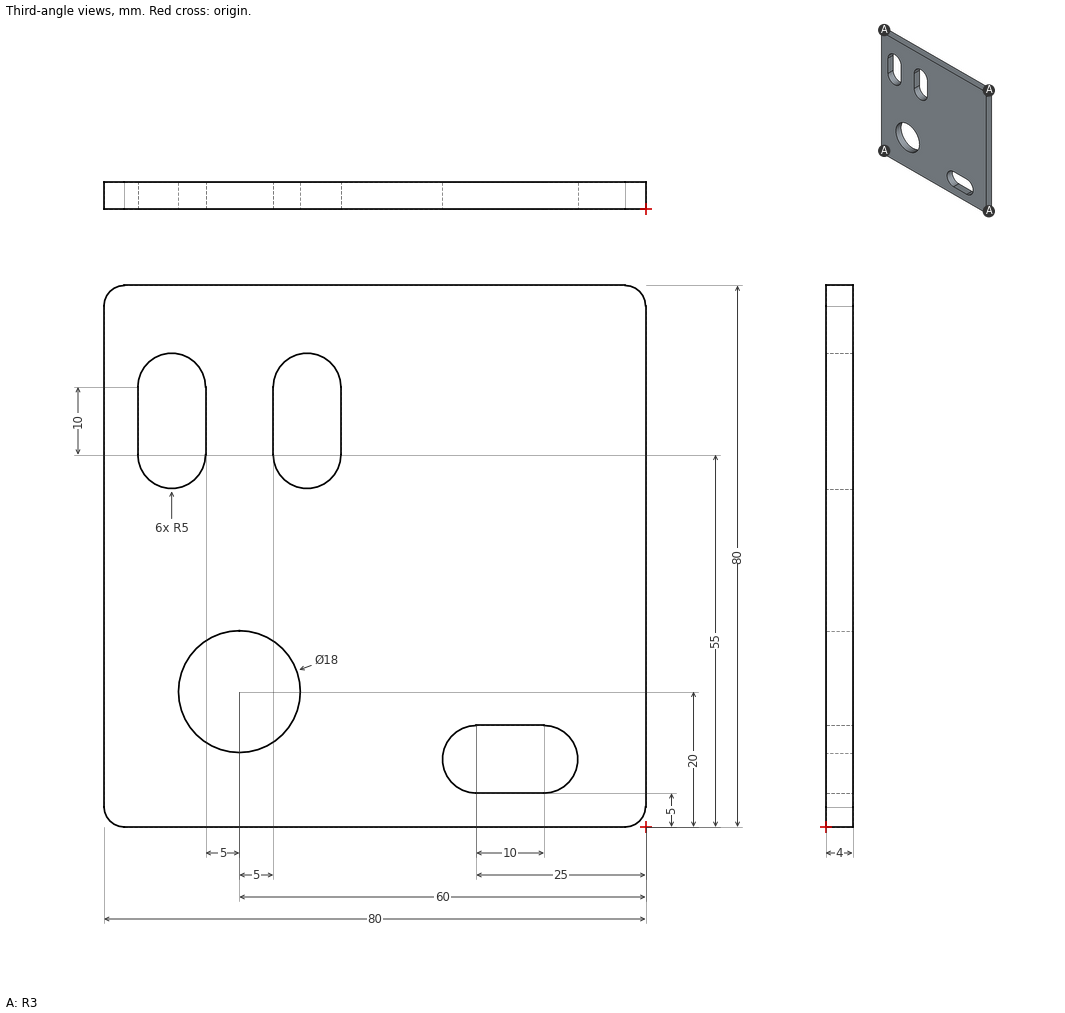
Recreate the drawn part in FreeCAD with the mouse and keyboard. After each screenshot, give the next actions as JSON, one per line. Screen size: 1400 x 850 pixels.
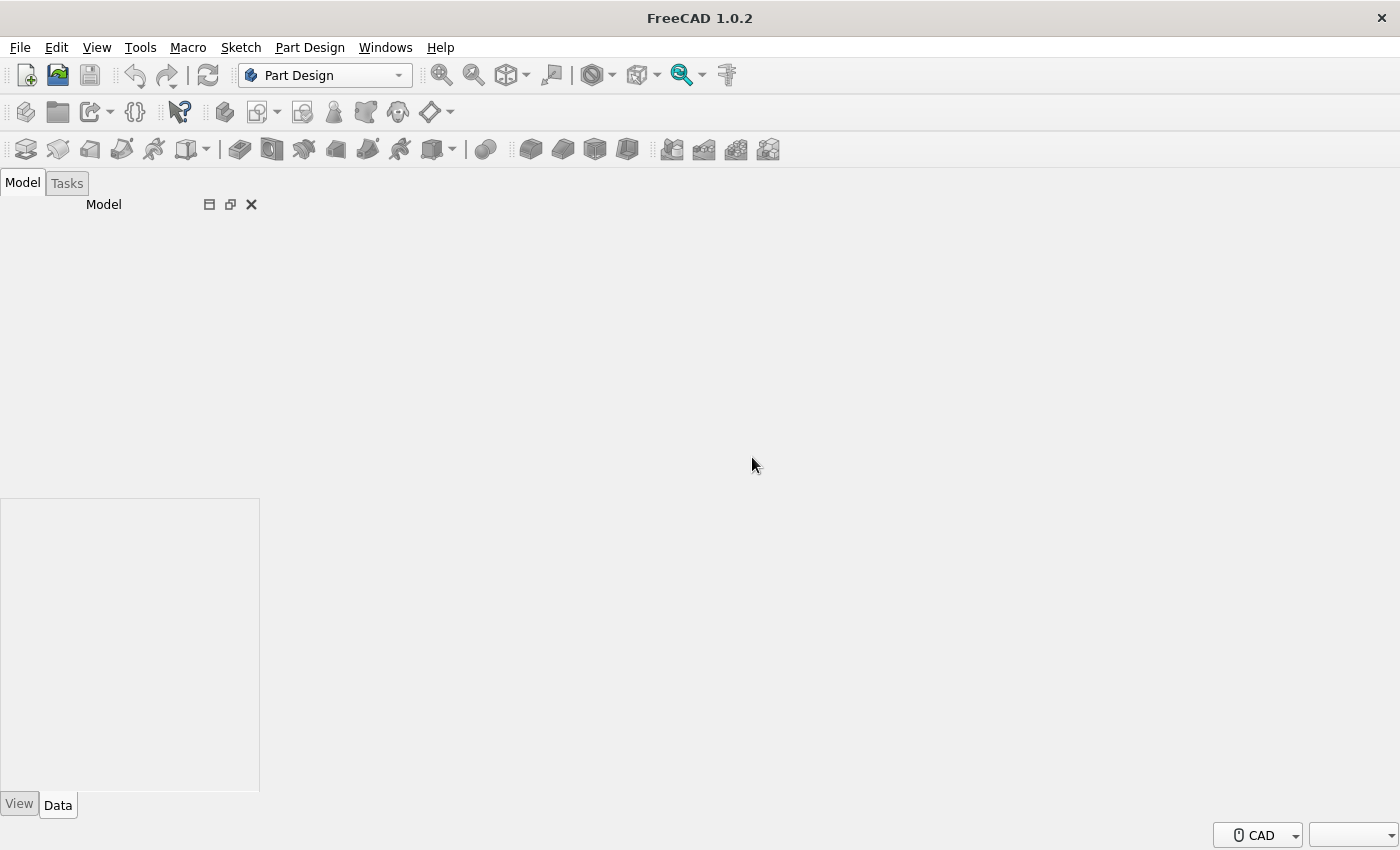
{"action": "left_click", "coordinate": [26, 76]}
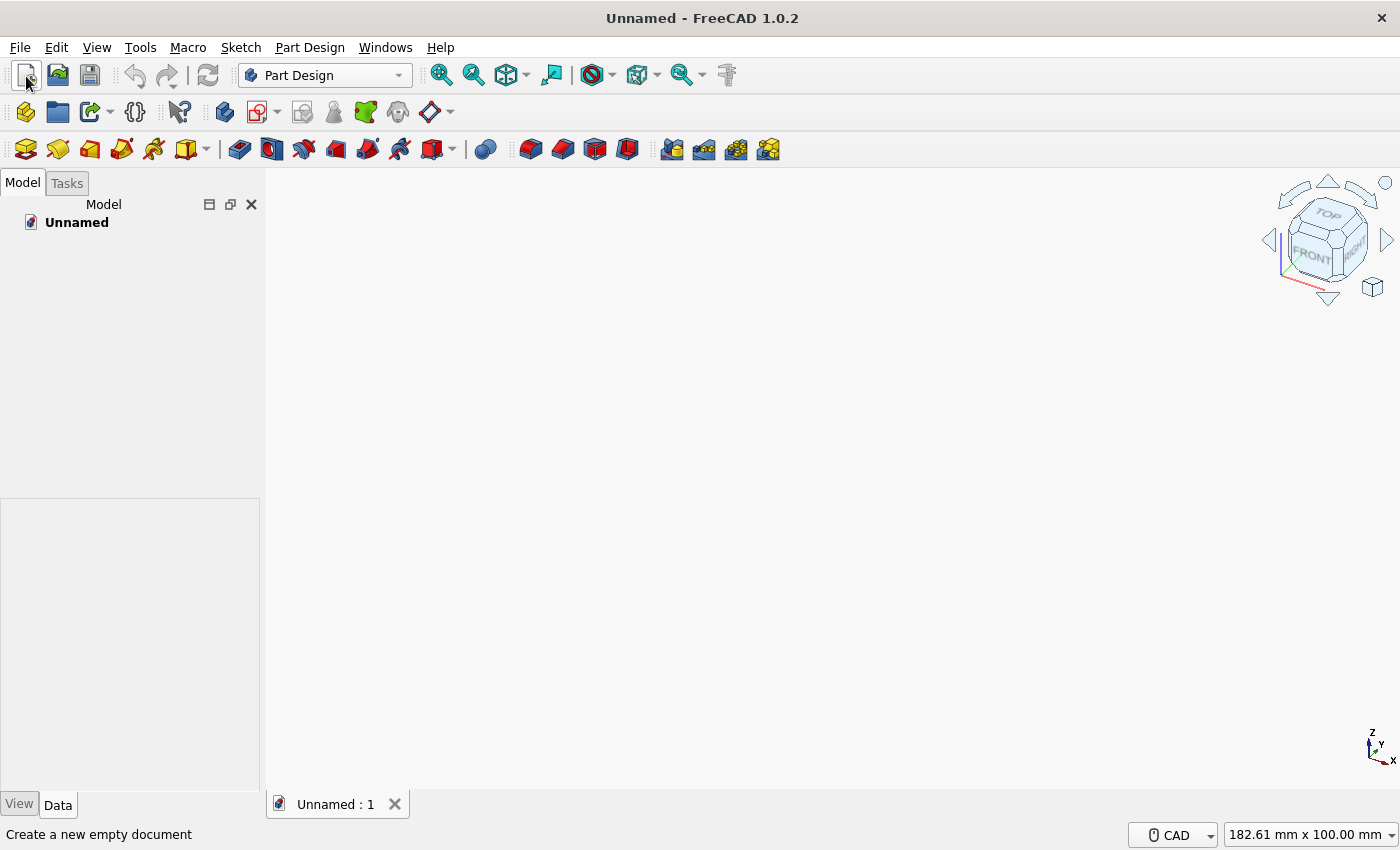
{"action": "left_click", "coordinate": [258, 112]}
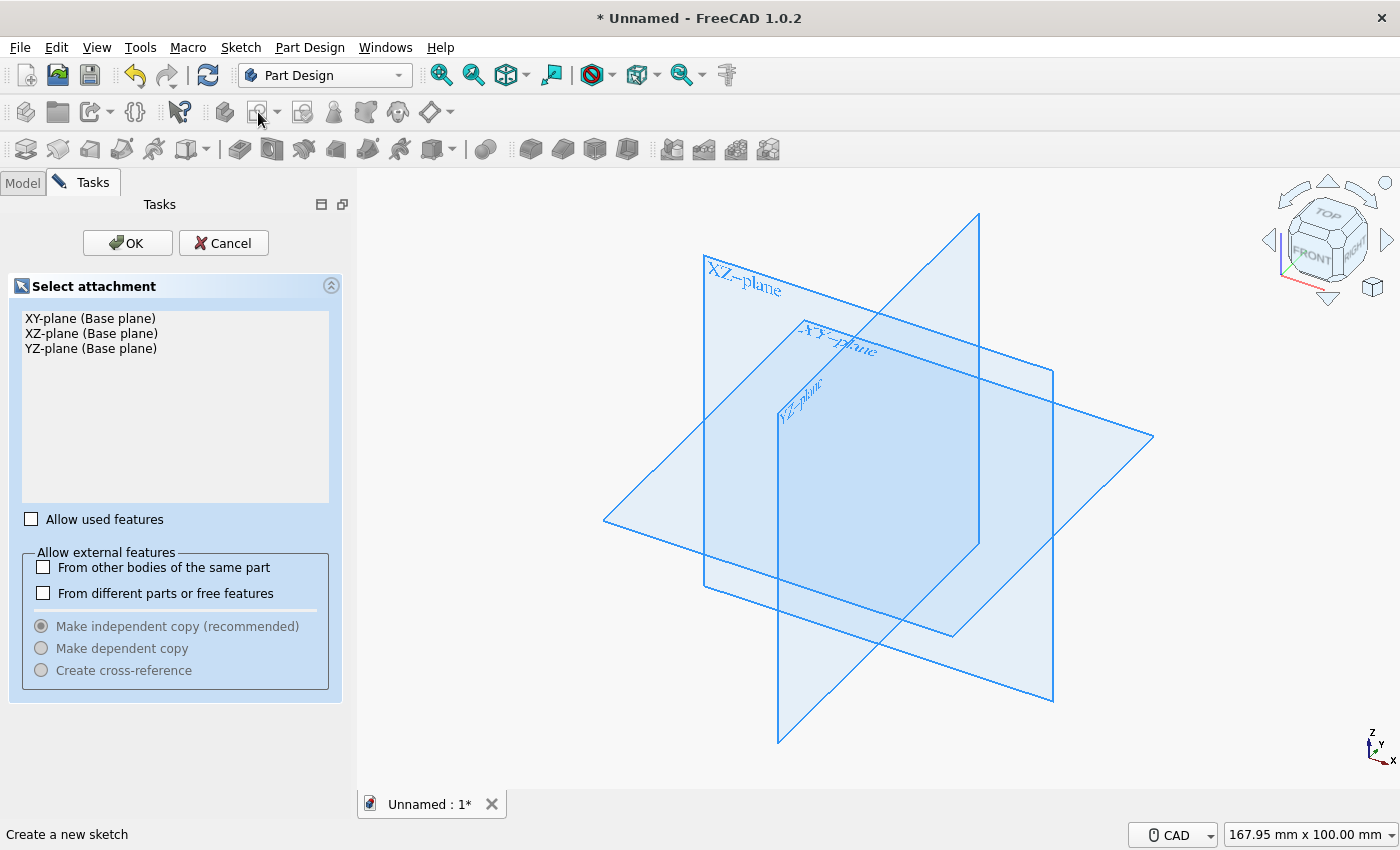
{"action": "left_click", "coordinate": [82, 334]}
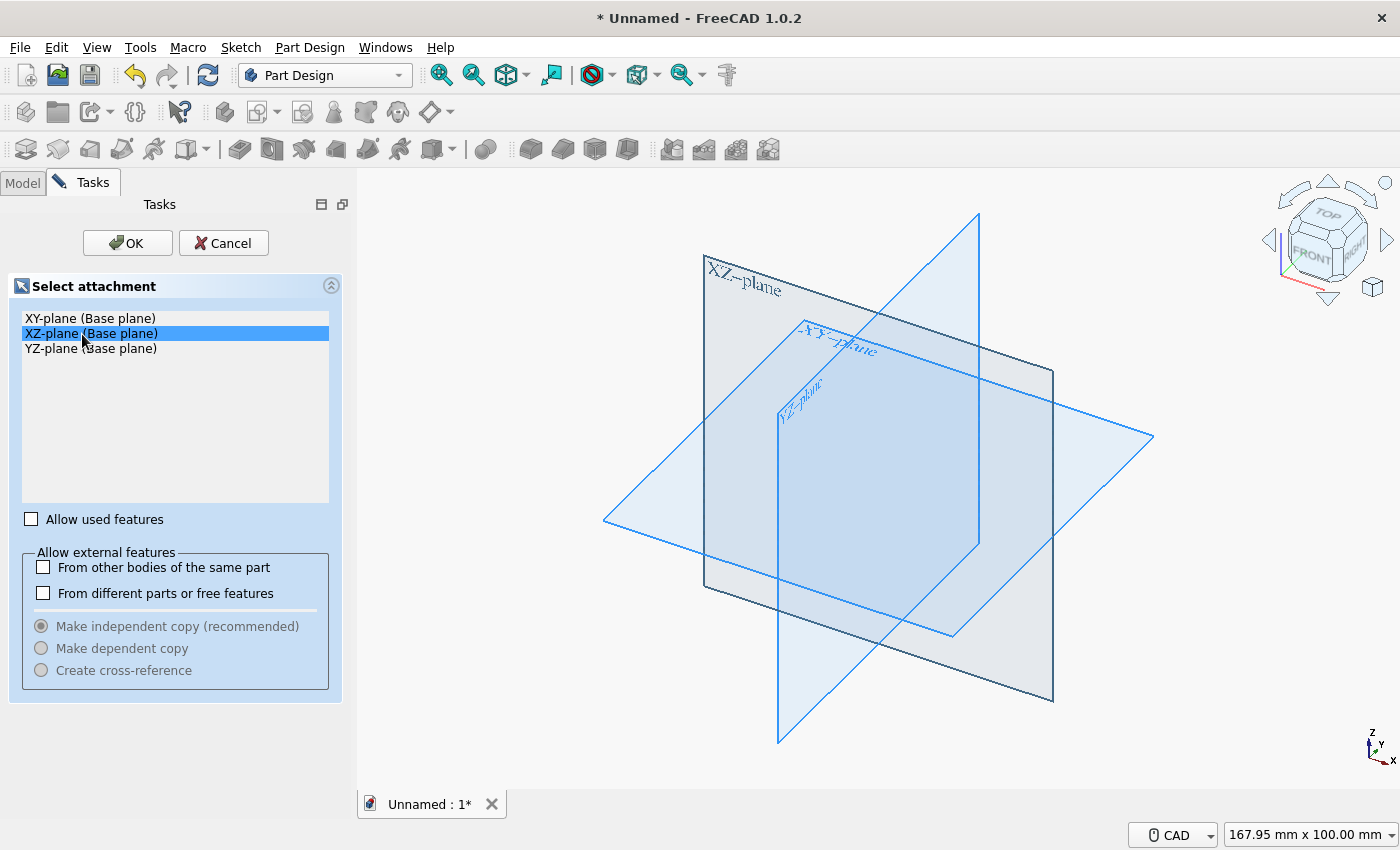
{"action": "left_click", "coordinate": [128, 243]}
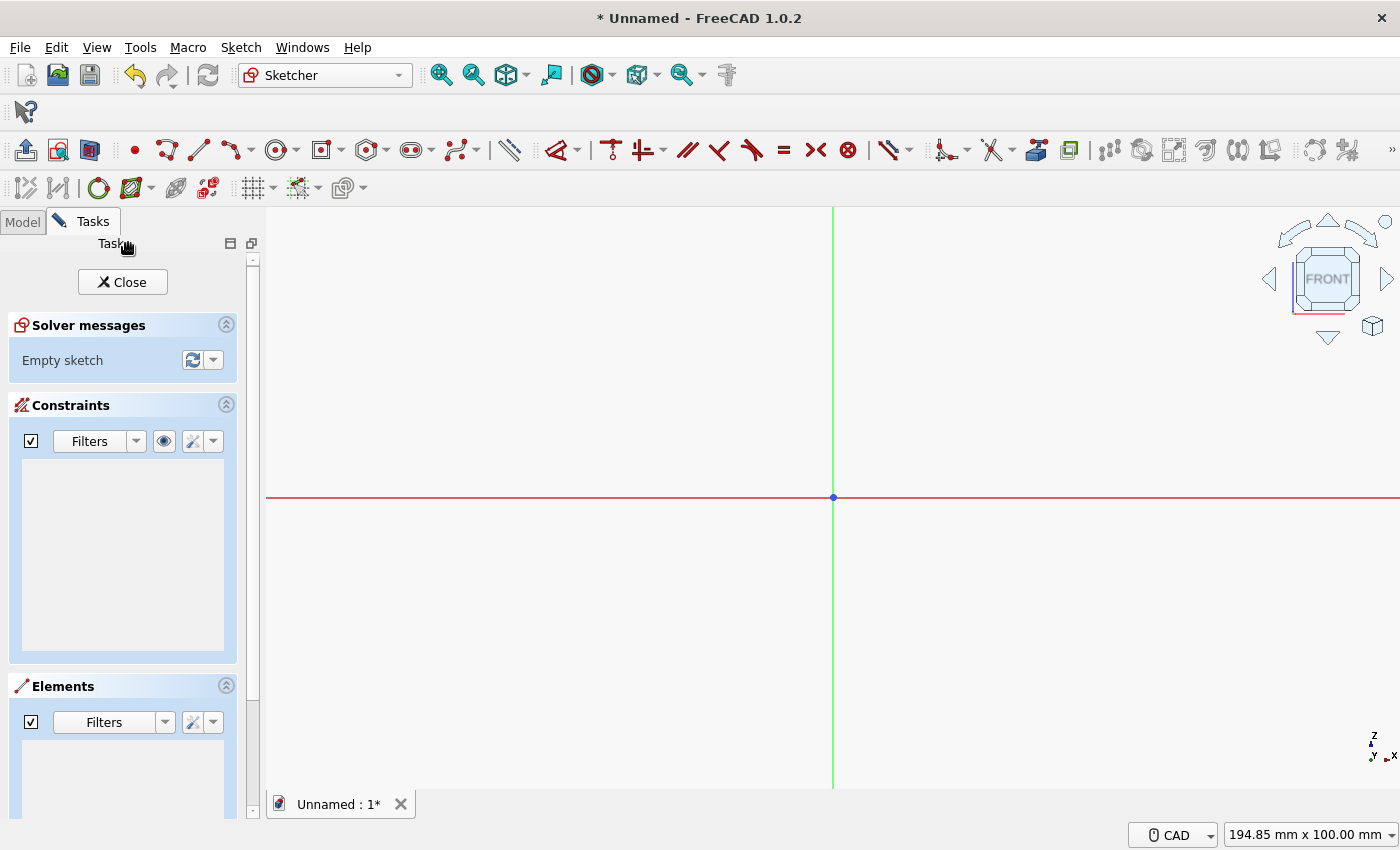
{"action": "scroll", "coordinate": [1099, 761], "scroll_direction": "down", "scroll_amount": 2}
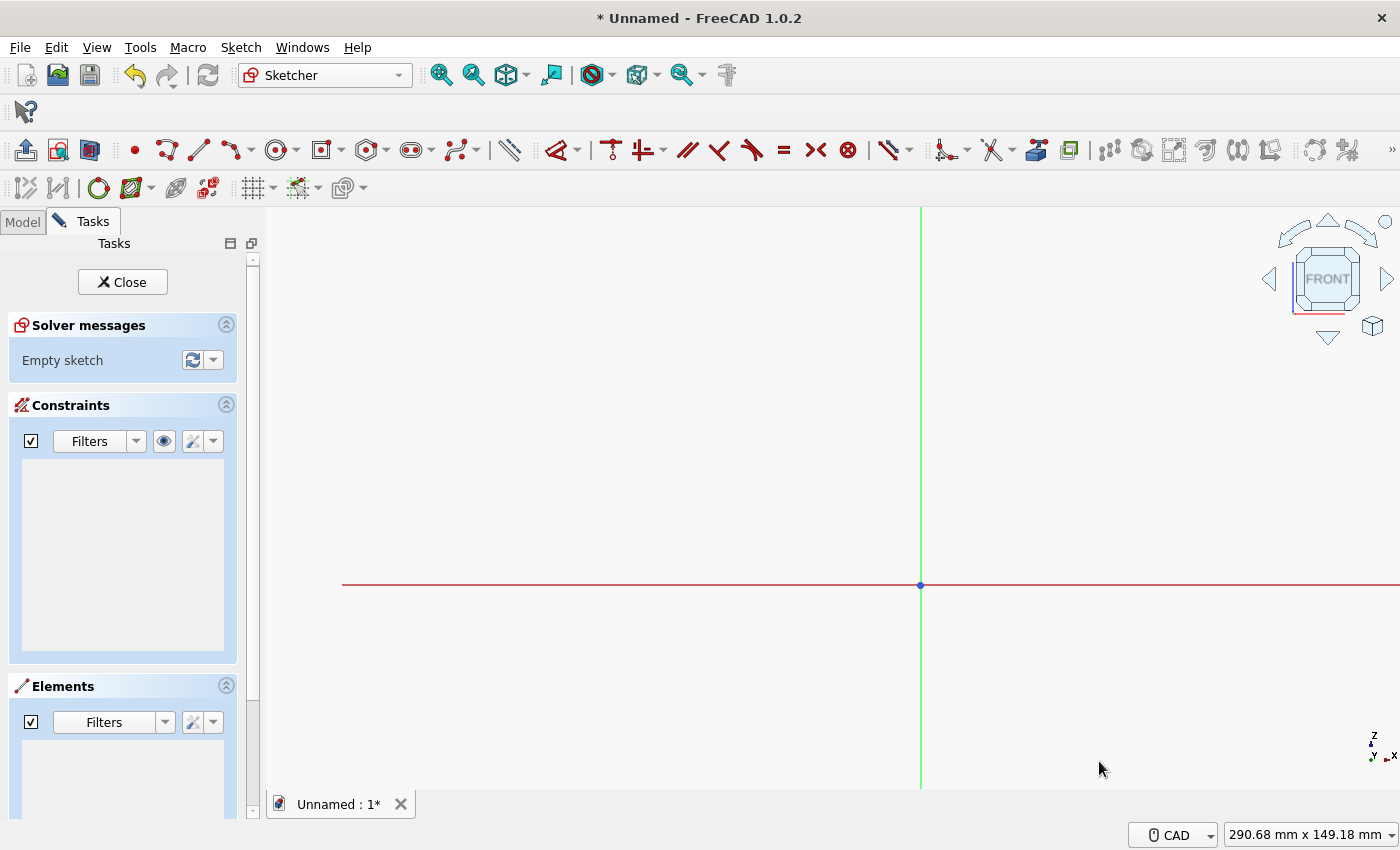
{"action": "left_click", "coordinate": [344, 150]}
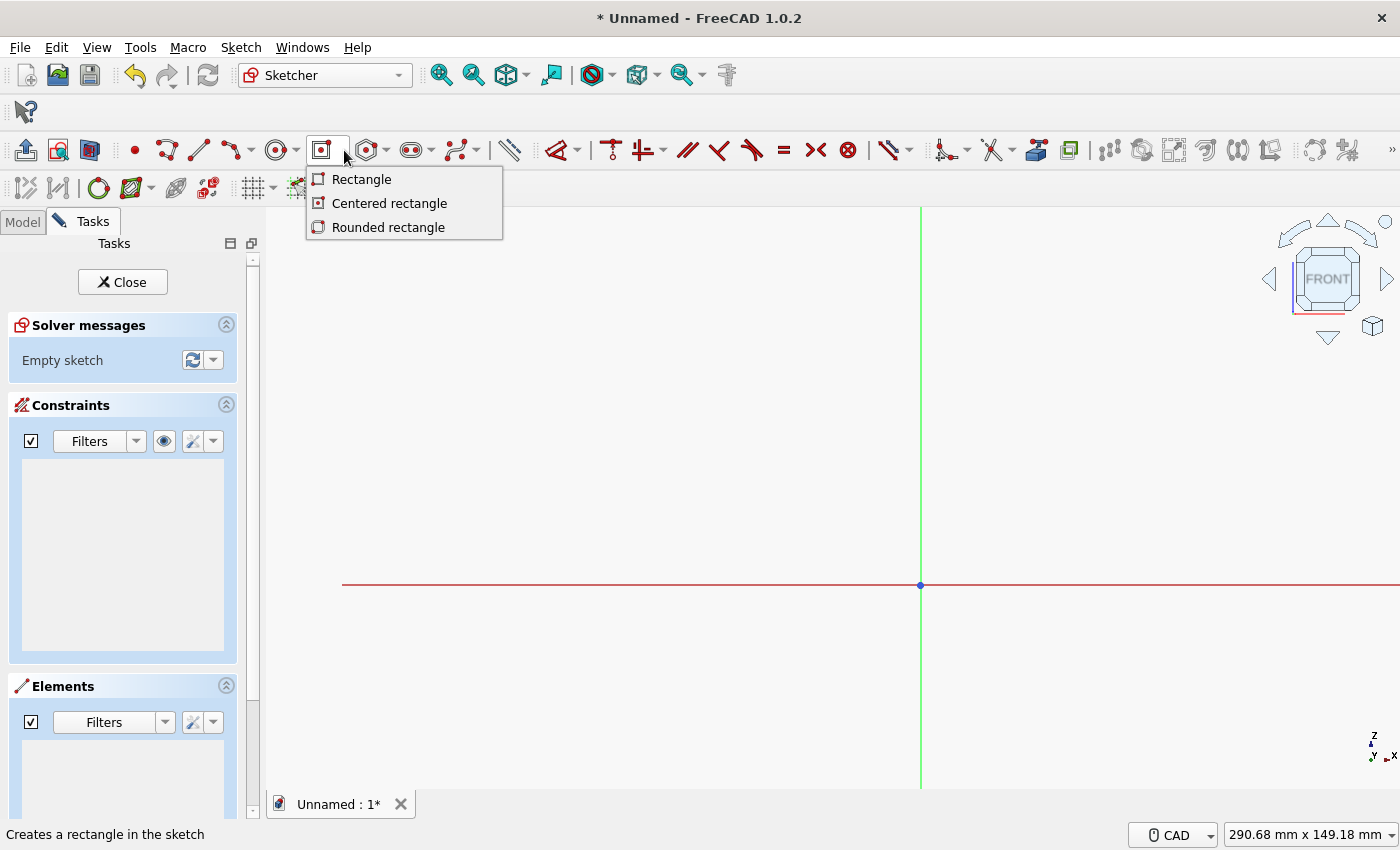
{"action": "left_click", "coordinate": [404, 179]}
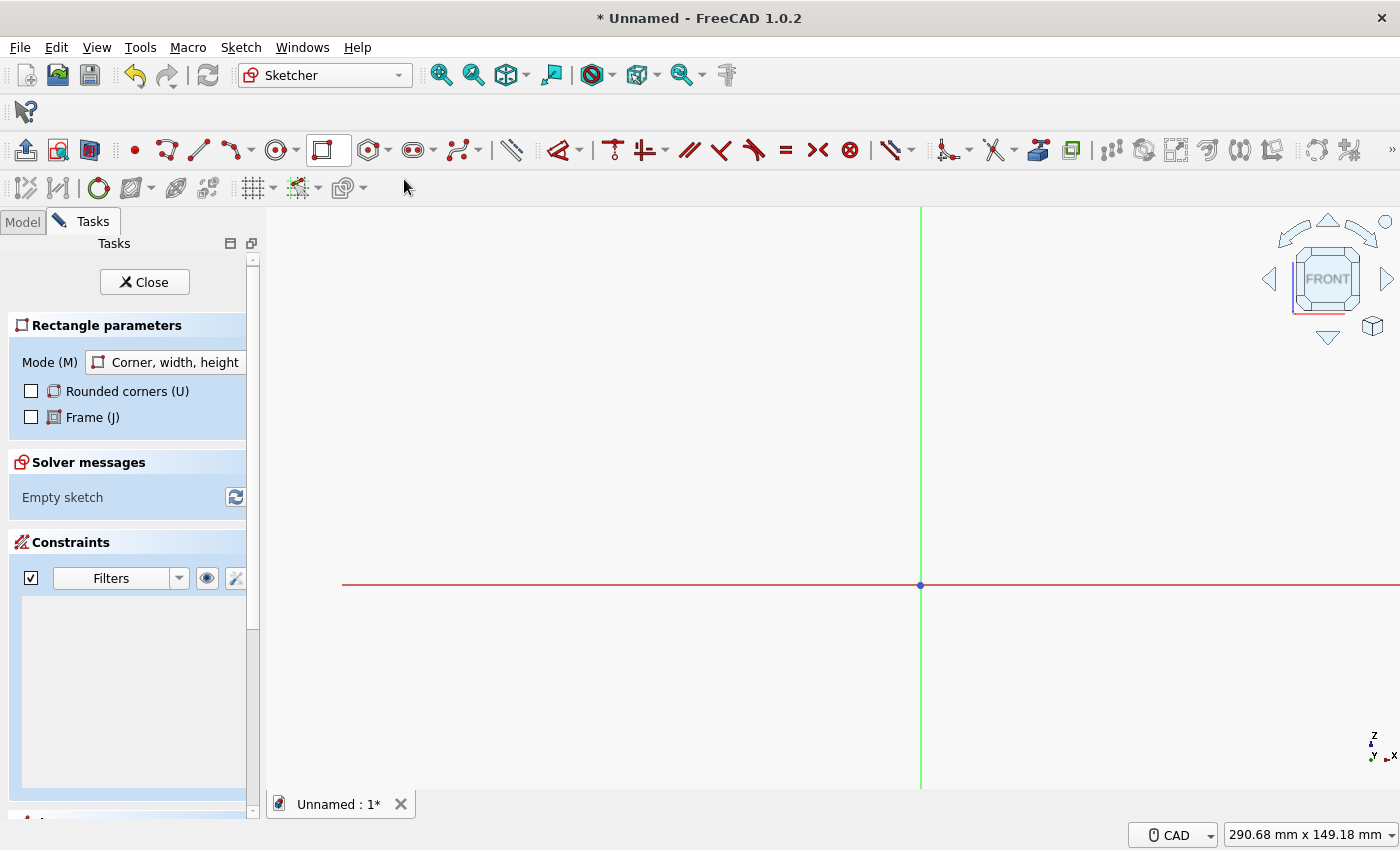
{"action": "left_click", "coordinate": [921, 585]}
{"action": "mouse_move", "coordinate": [609, 273]}